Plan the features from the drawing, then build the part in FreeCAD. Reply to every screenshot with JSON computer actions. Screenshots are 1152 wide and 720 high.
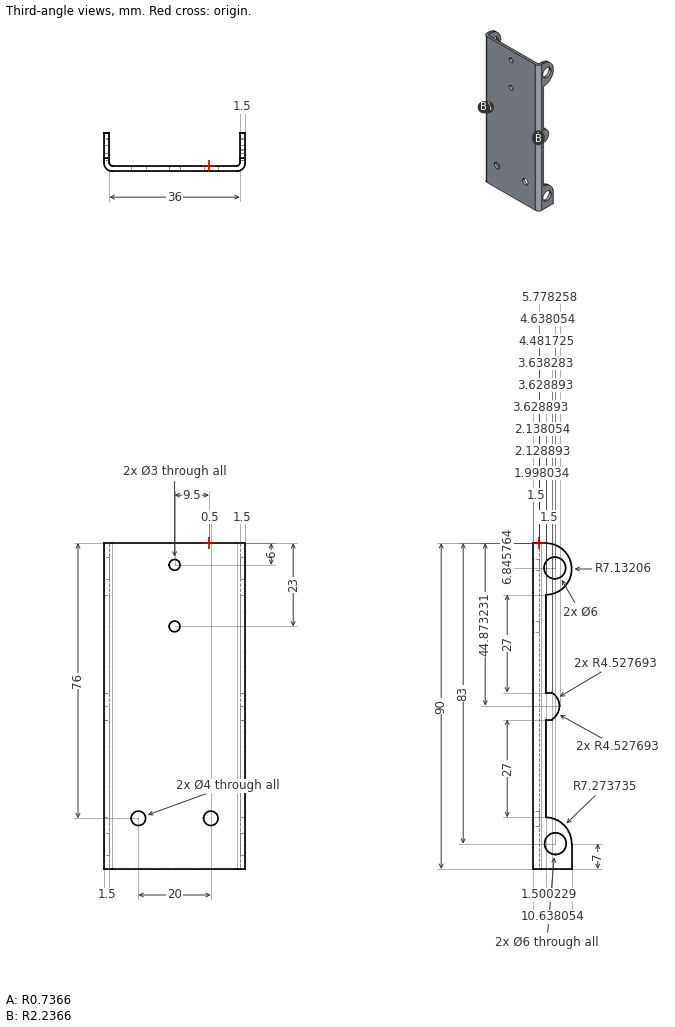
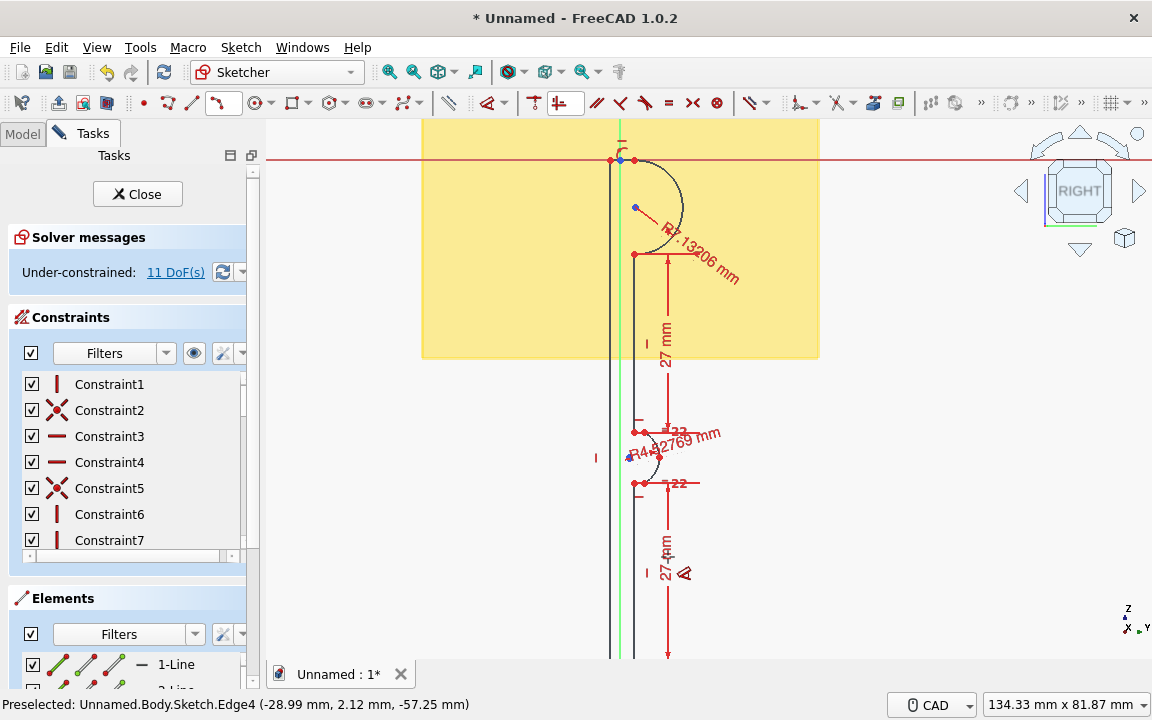
{"action": "scroll", "coordinate": [610, 577], "scroll_direction": "up", "scroll_amount": 2}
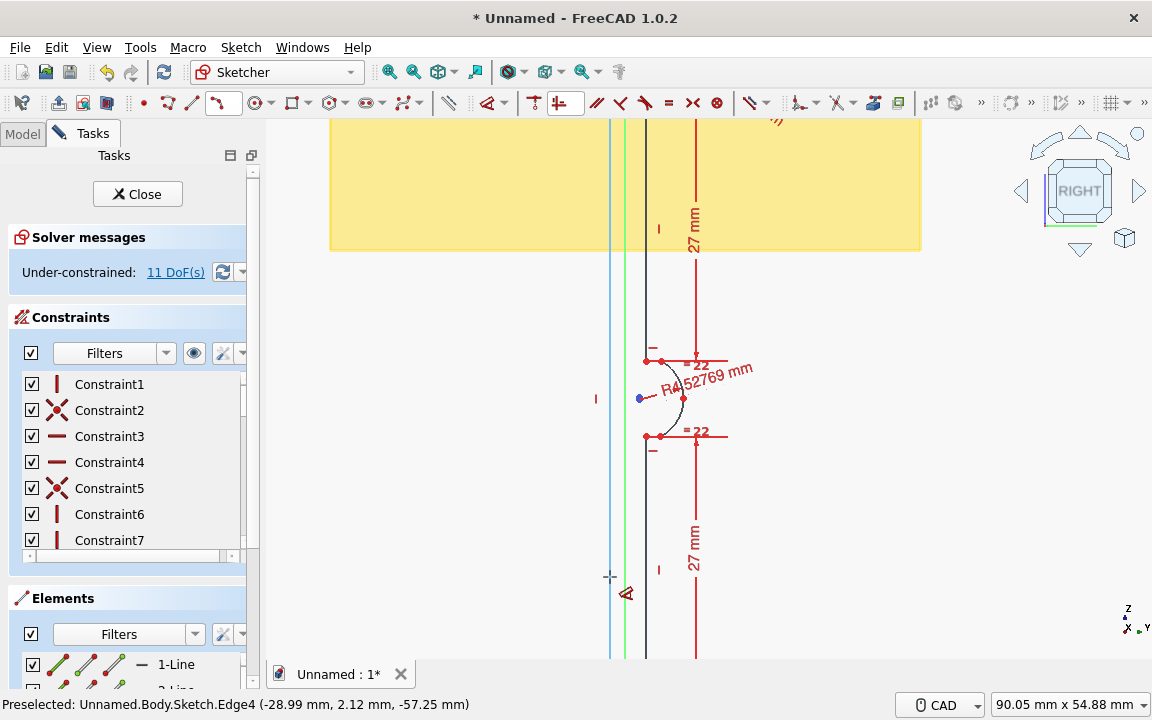
{"action": "left_click", "coordinate": [610, 576]}
{"action": "left_click", "coordinate": [576, 389]}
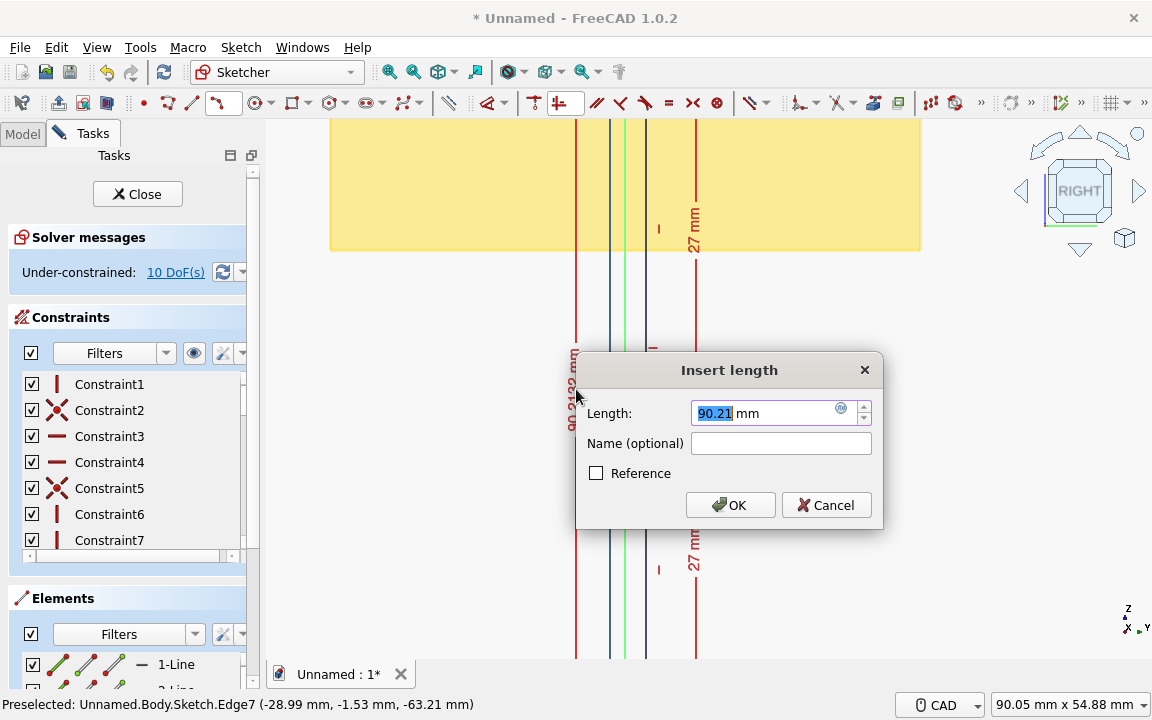
{"action": "type", "text": "90"}
{"action": "key", "text": "Return"}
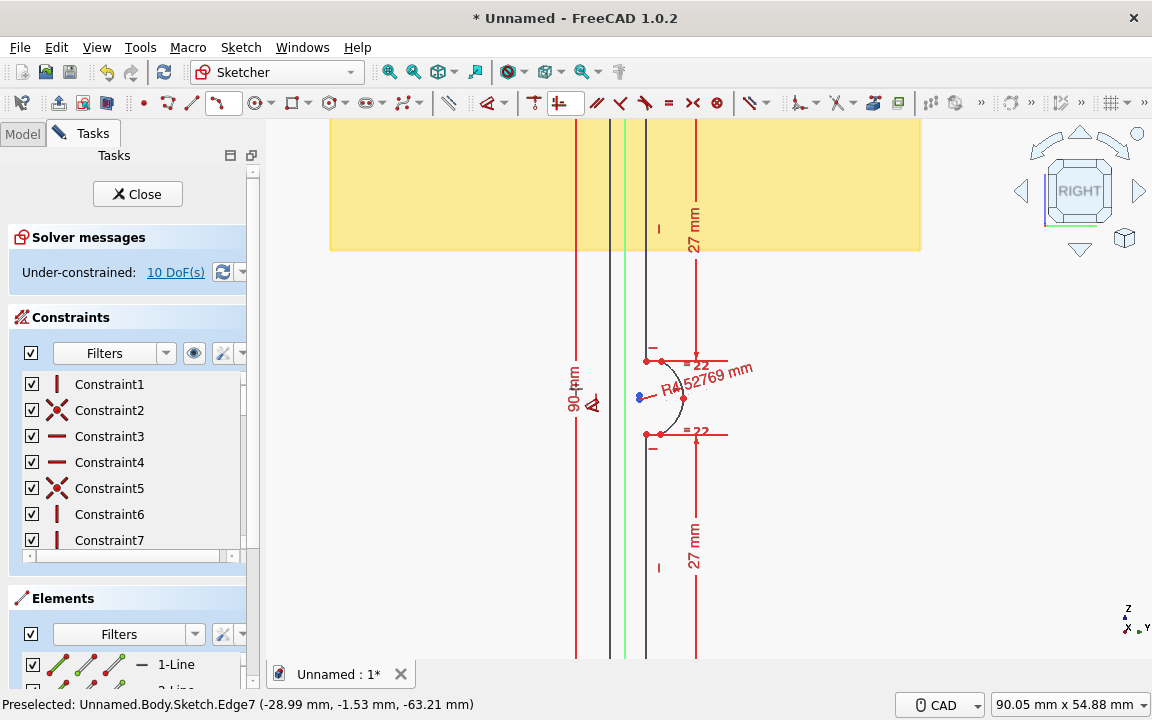
{"action": "scroll", "coordinate": [654, 361], "scroll_direction": "up", "scroll_amount": 5}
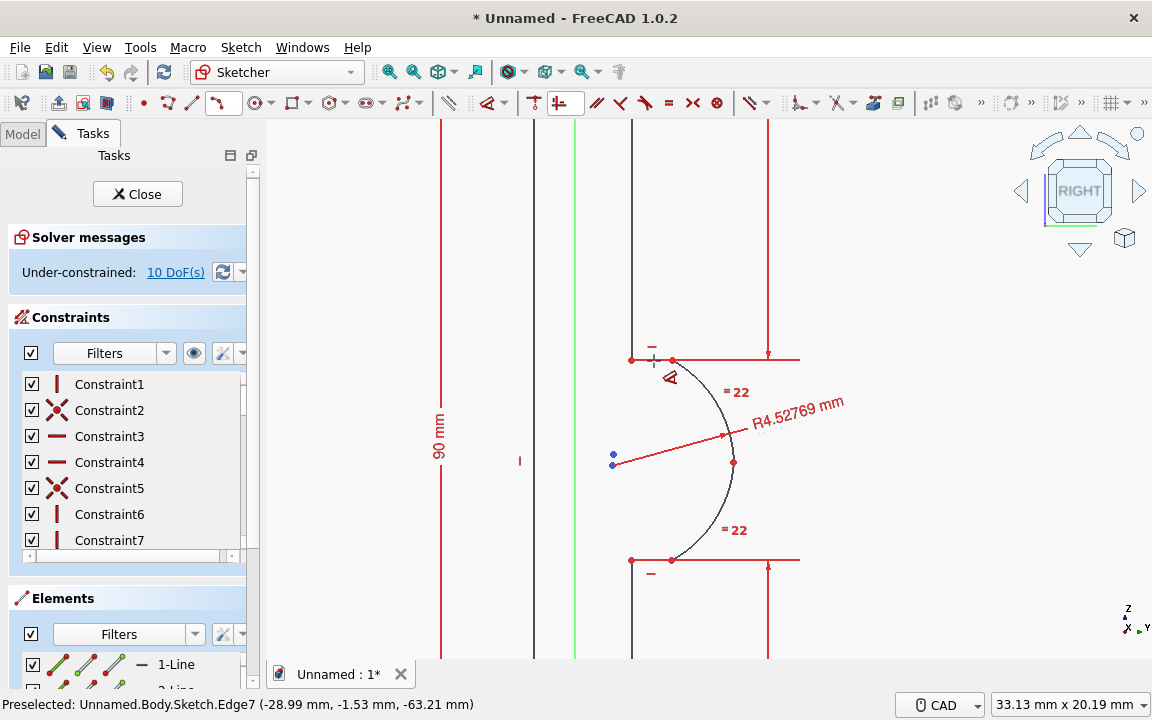
{"action": "left_click", "coordinate": [652, 360]}
{"action": "left_click", "coordinate": [652, 326]}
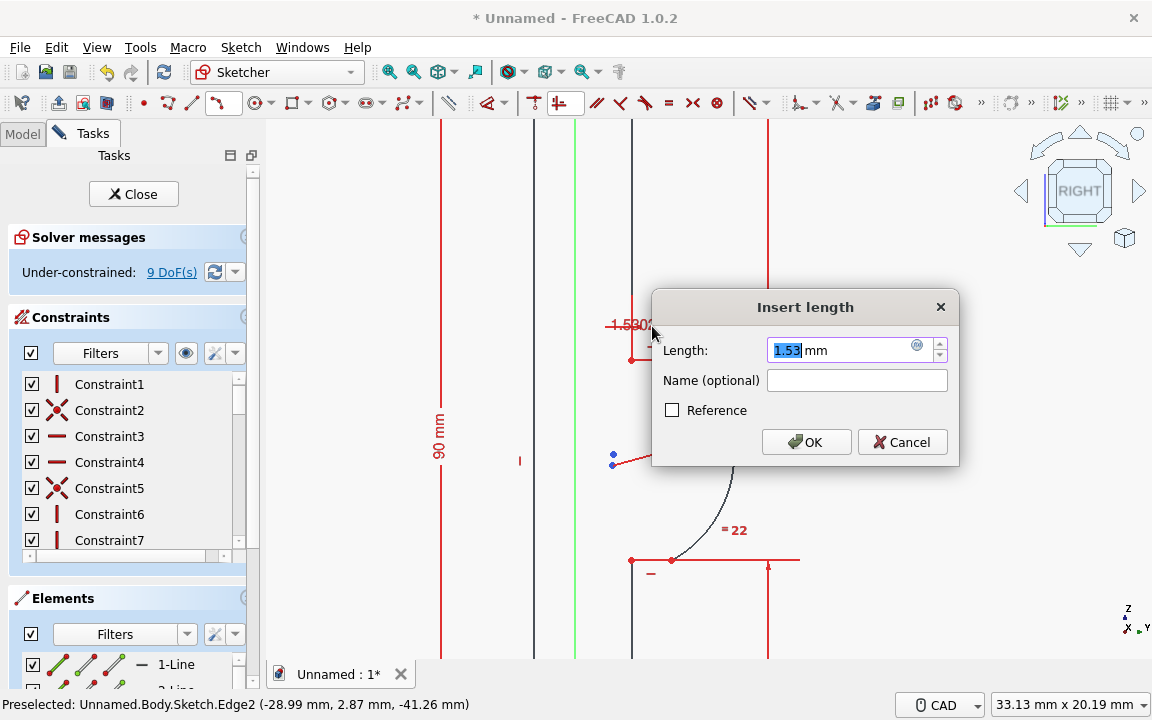
{"action": "type", "text": "1.5"}
{"action": "key", "text": "Return"}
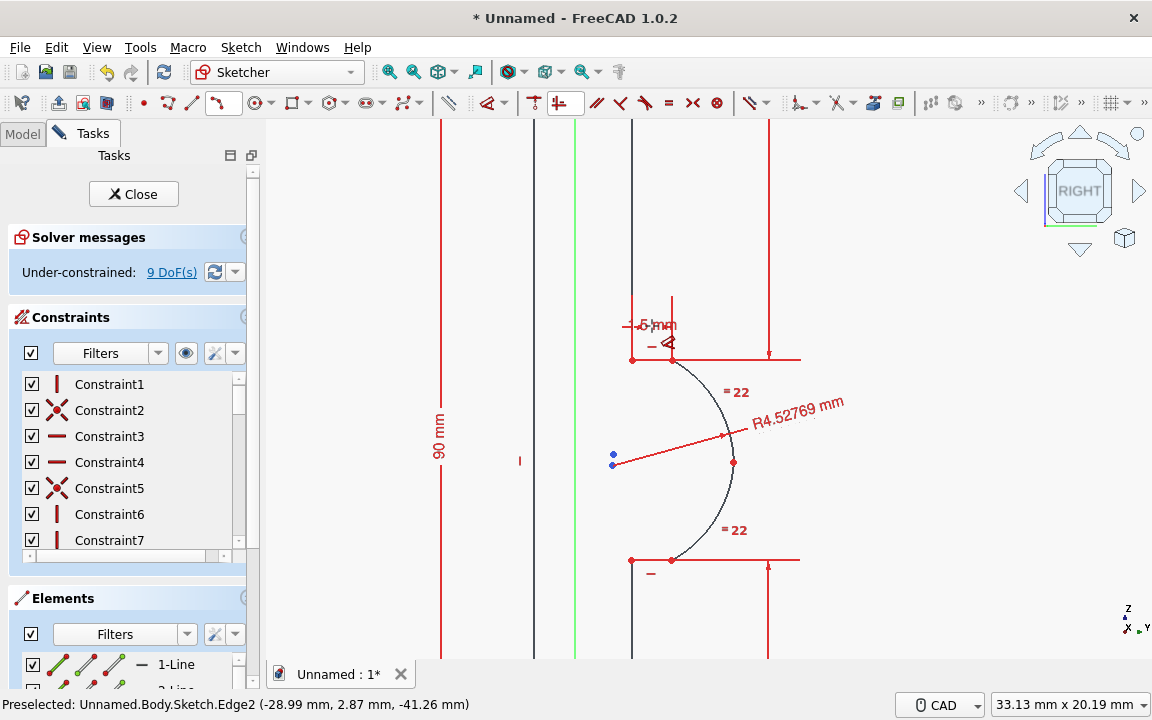
{"action": "scroll", "coordinate": [635, 378], "scroll_direction": "down", "scroll_amount": 10}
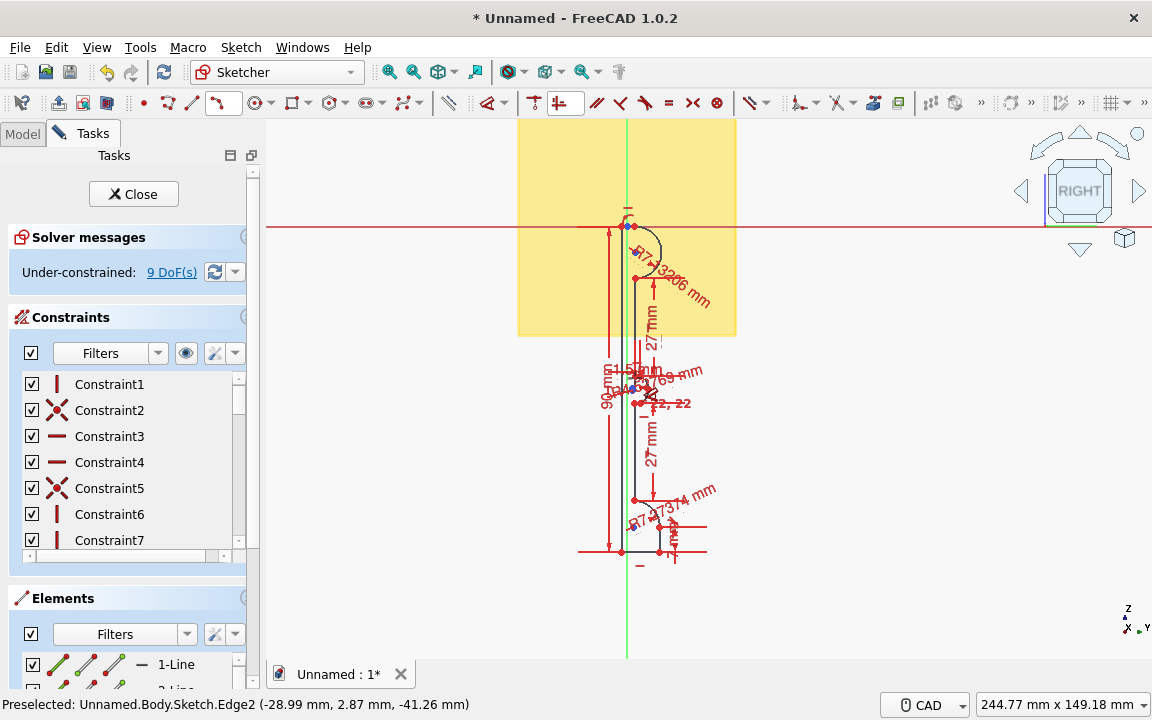
{"action": "scroll", "coordinate": [622, 552], "scroll_direction": "up", "scroll_amount": 10}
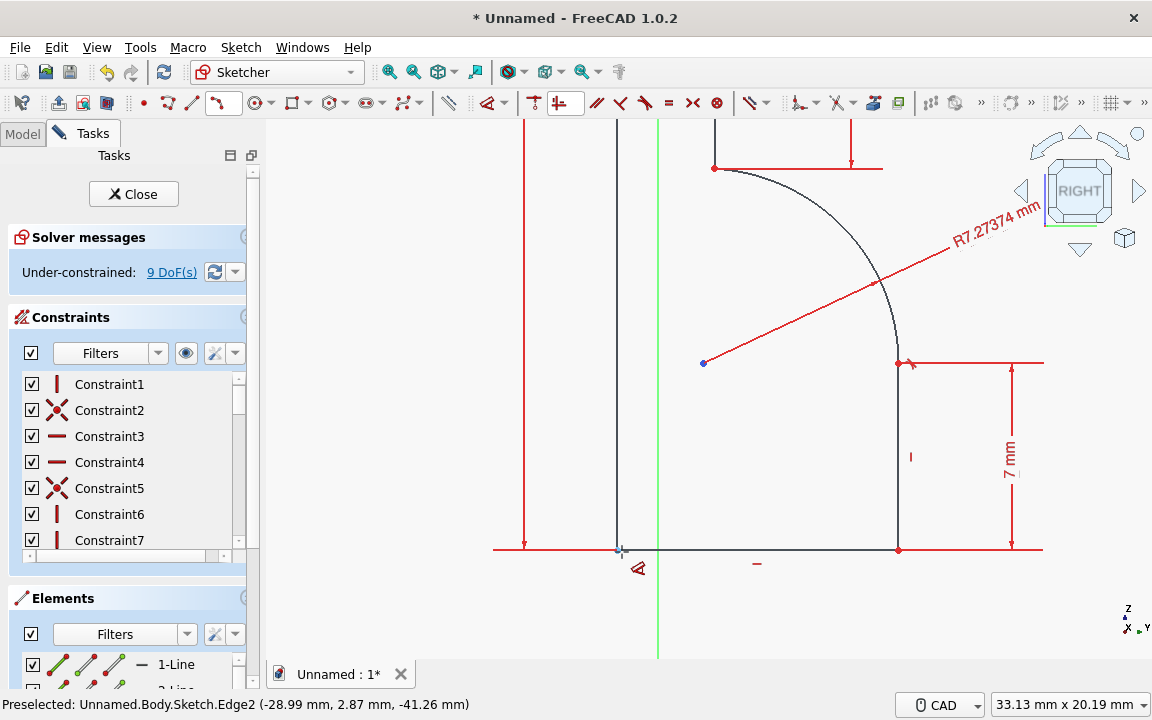
{"action": "left_click", "coordinate": [617, 550]}
{"action": "left_click", "coordinate": [638, 584]}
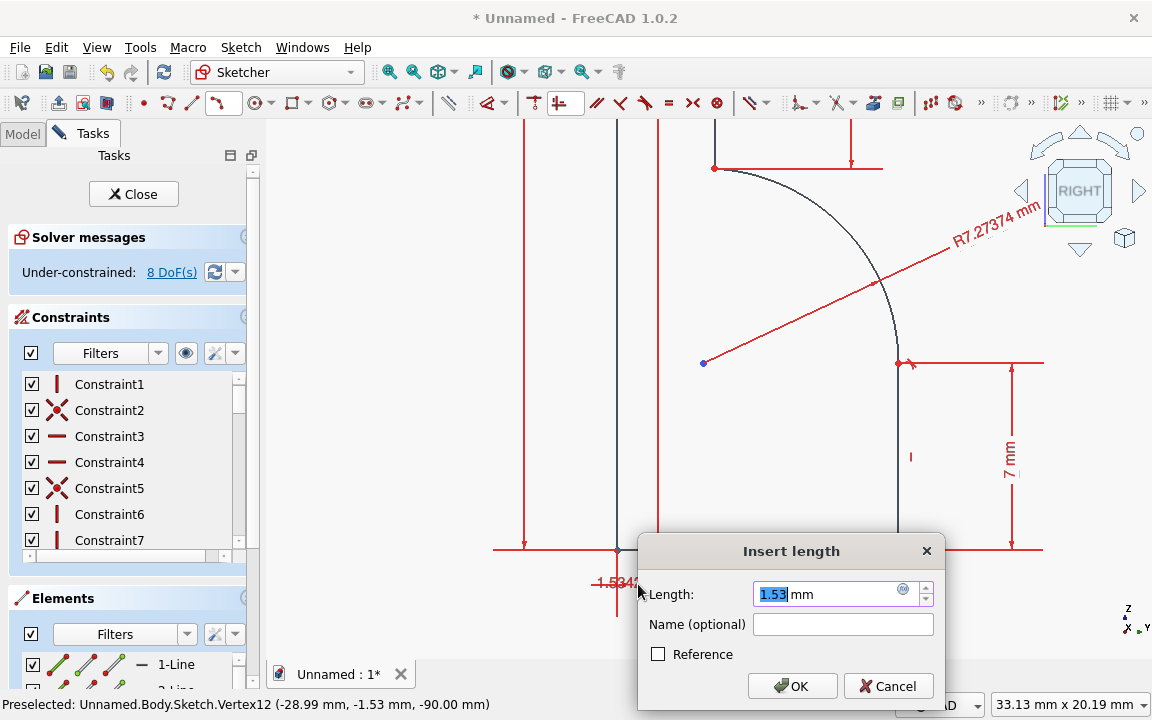
{"action": "type", "text": "1.5"}
{"action": "key", "text": "Return"}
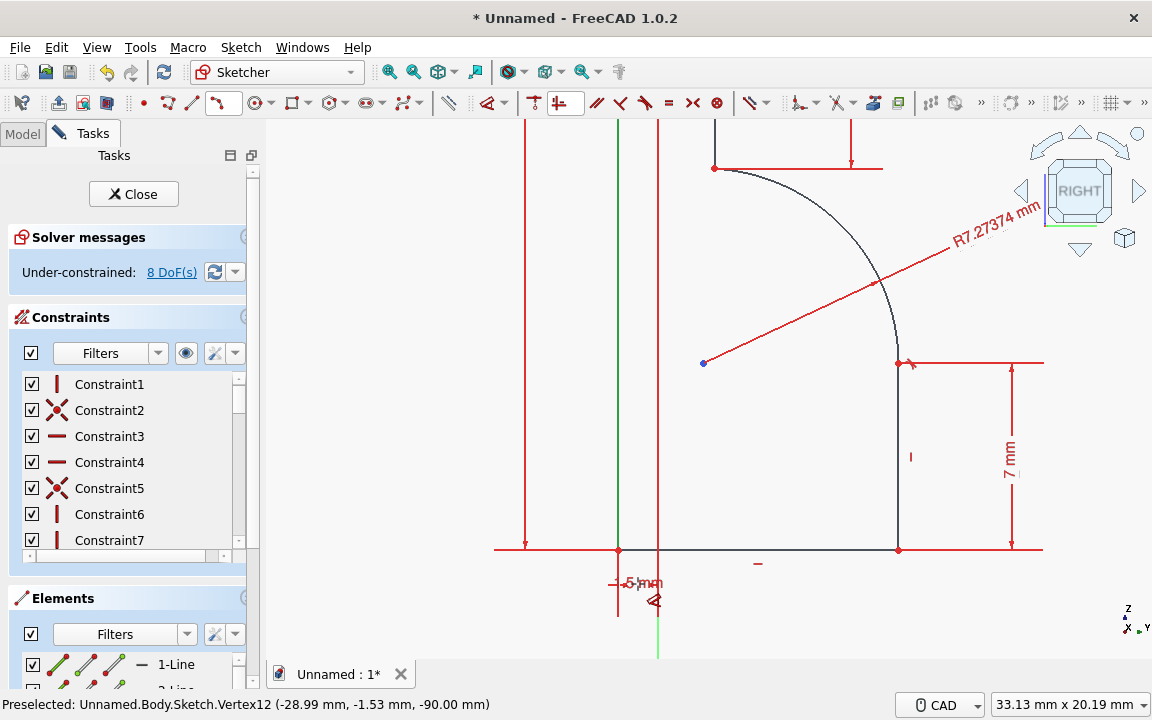
{"action": "scroll", "coordinate": [622, 552], "scroll_direction": "down", "scroll_amount": 10}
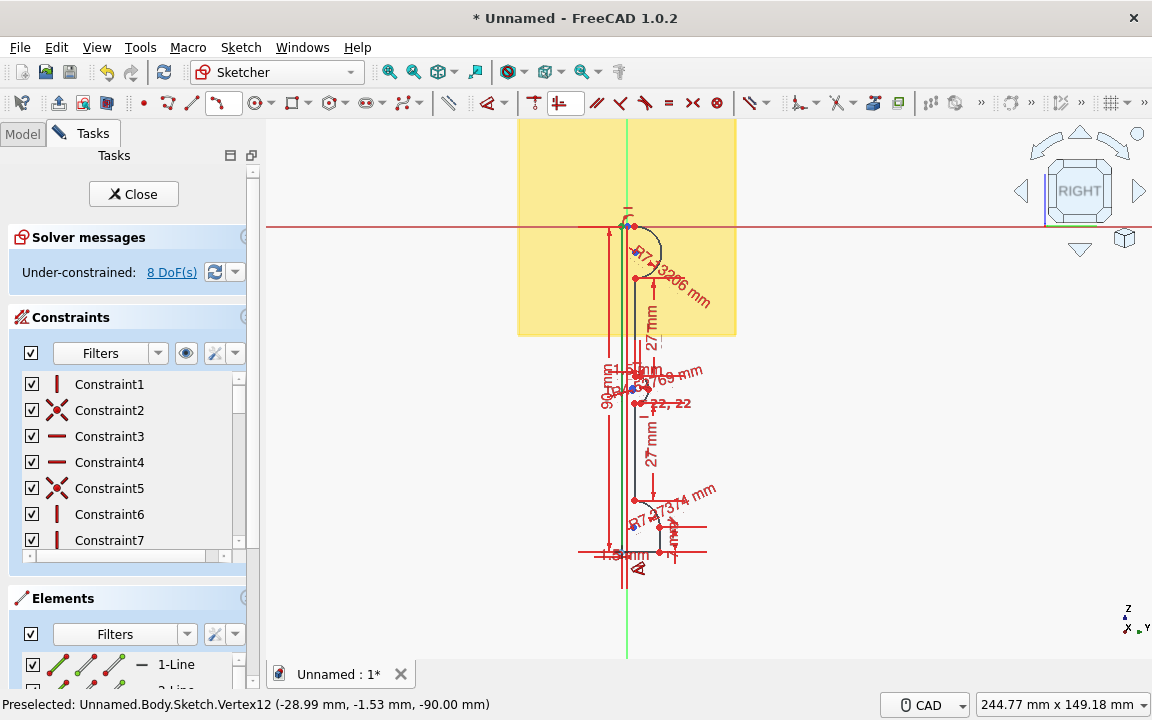
{"action": "scroll", "coordinate": [639, 403], "scroll_direction": "up", "scroll_amount": 11}